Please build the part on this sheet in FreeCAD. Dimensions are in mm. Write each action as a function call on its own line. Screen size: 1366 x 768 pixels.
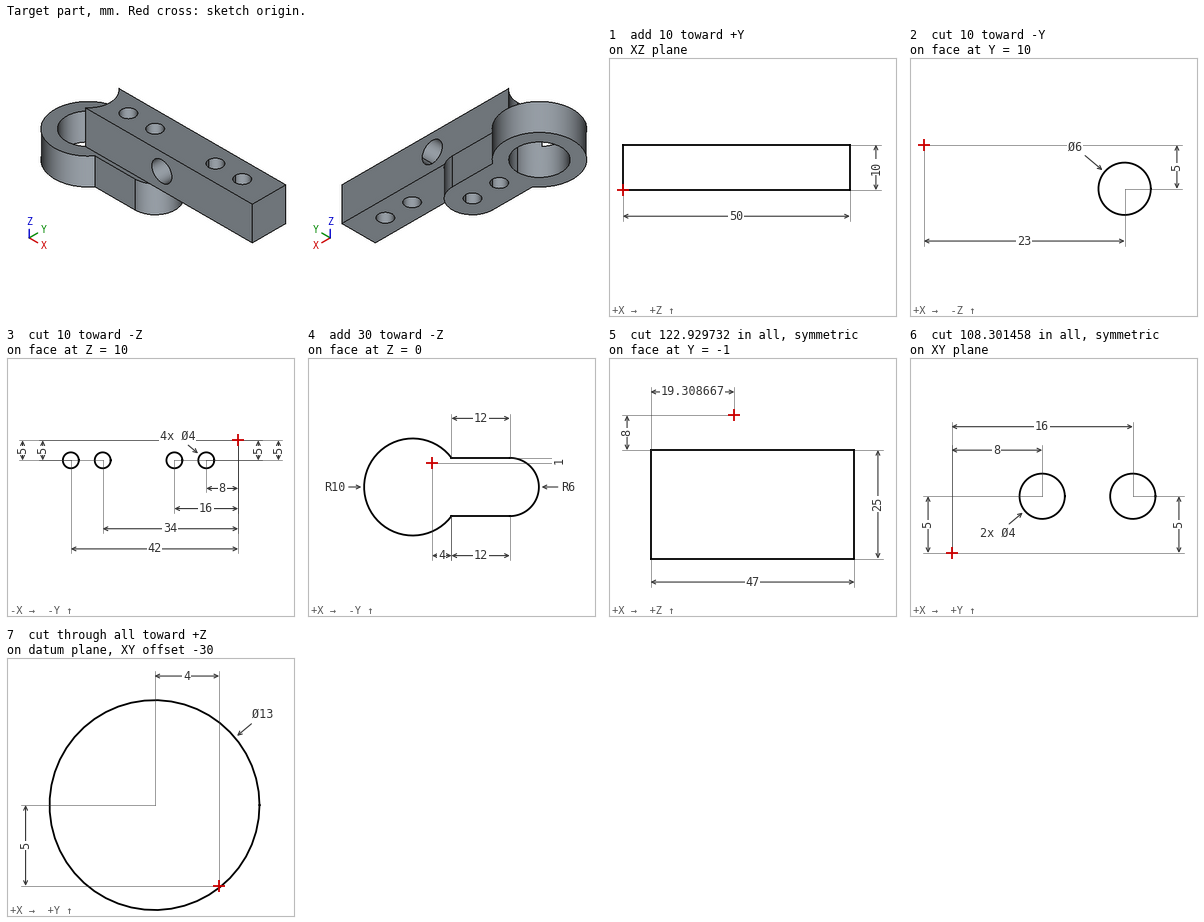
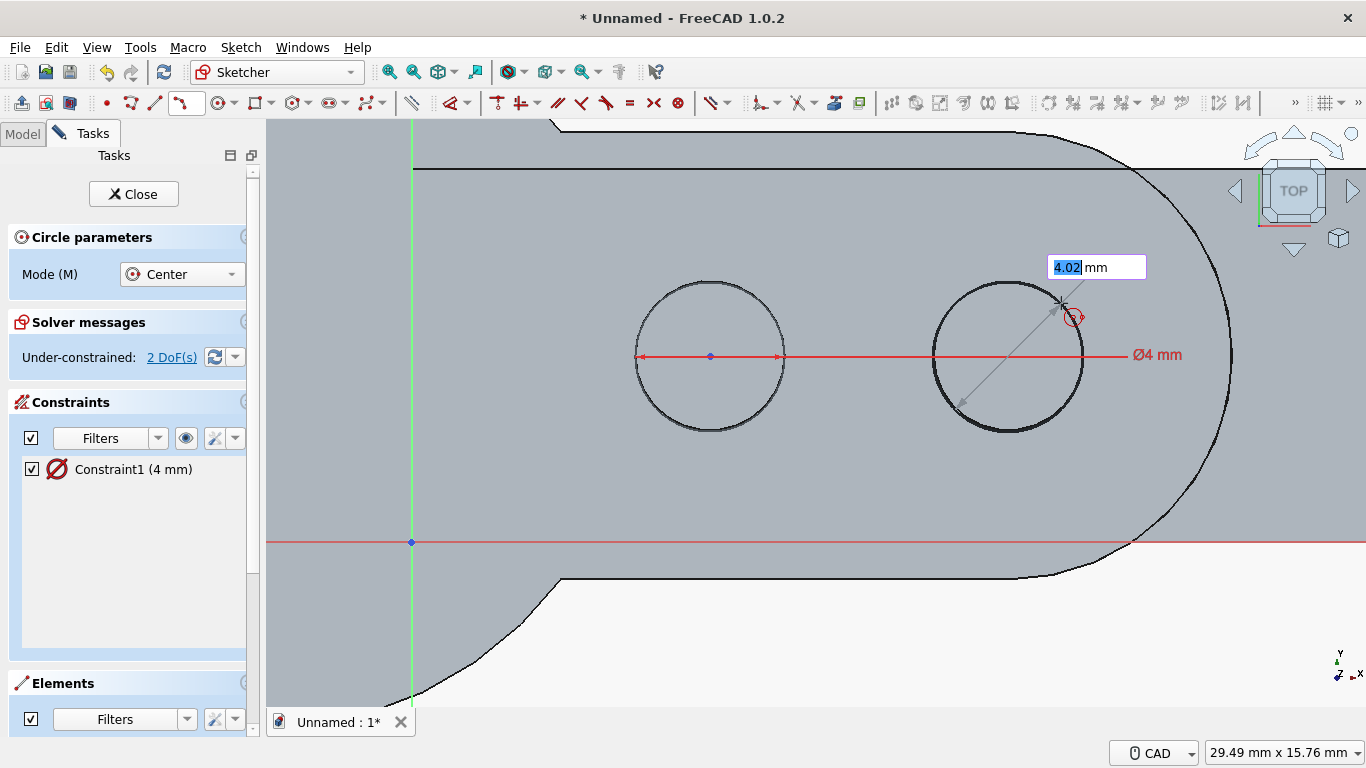
text(4)
key(Return)
key(Escape)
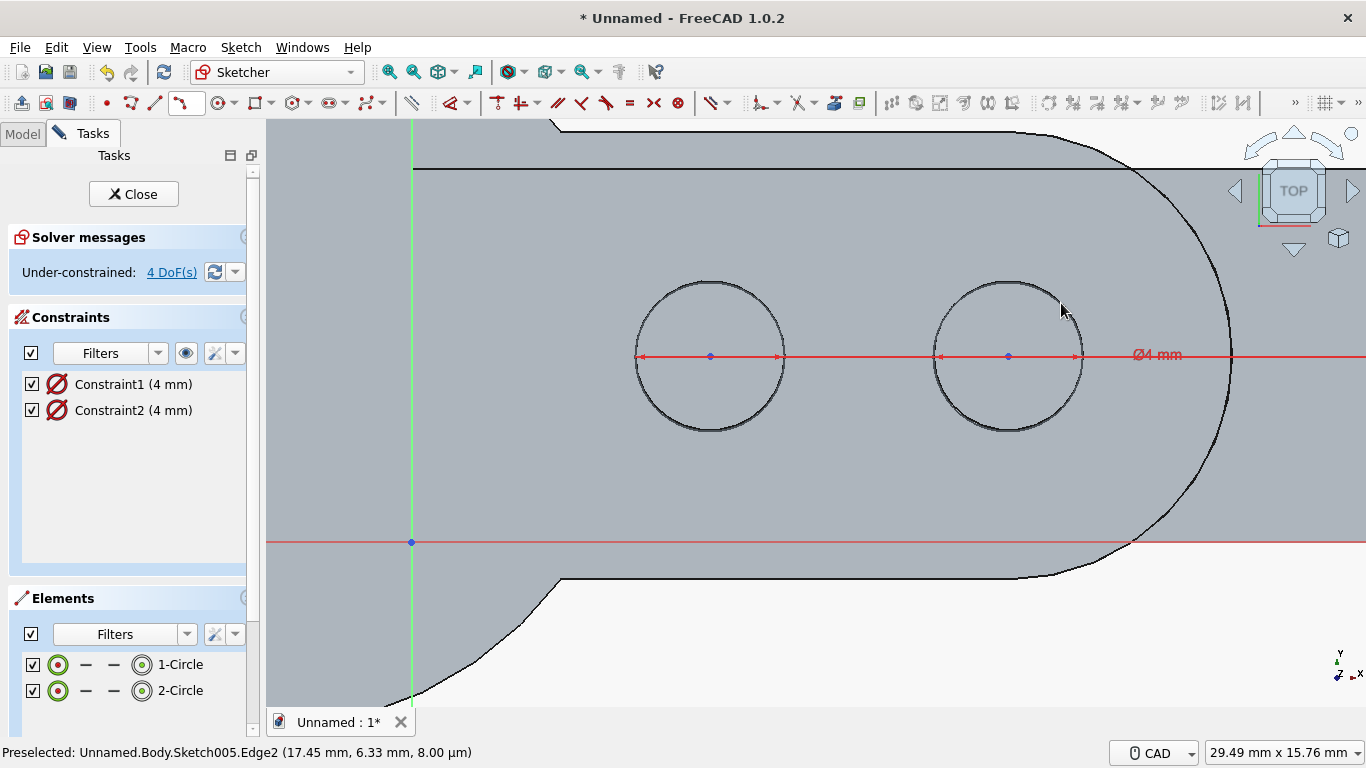
key(d)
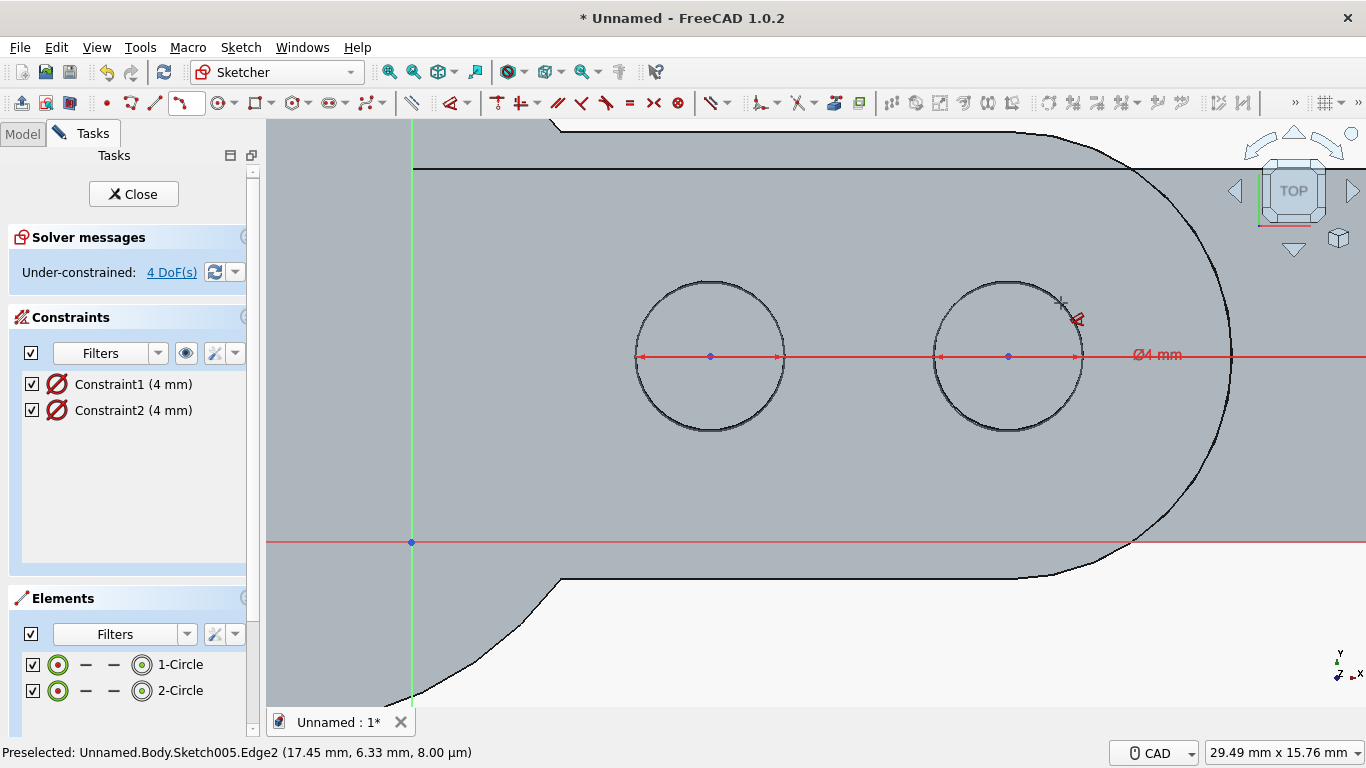
click(710, 357)
click(561, 576)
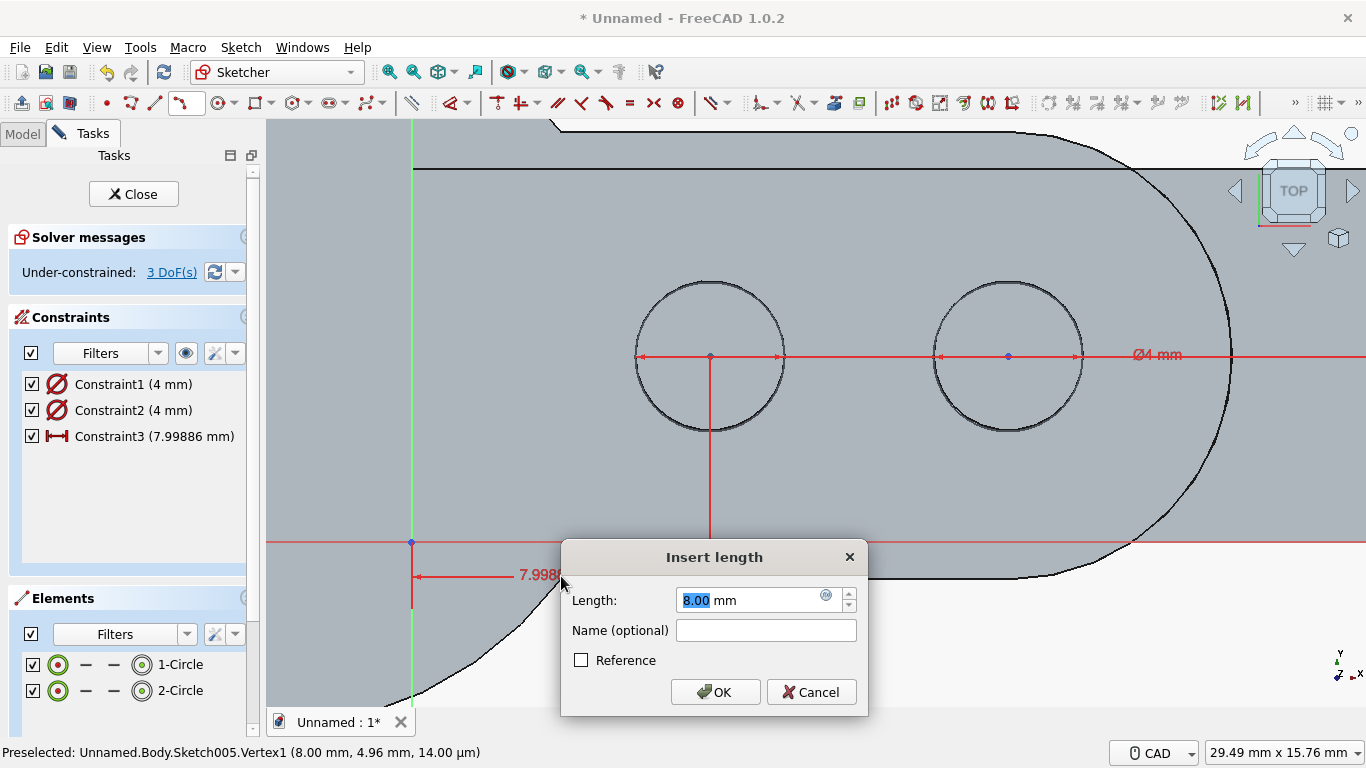
text(8)
key(Return)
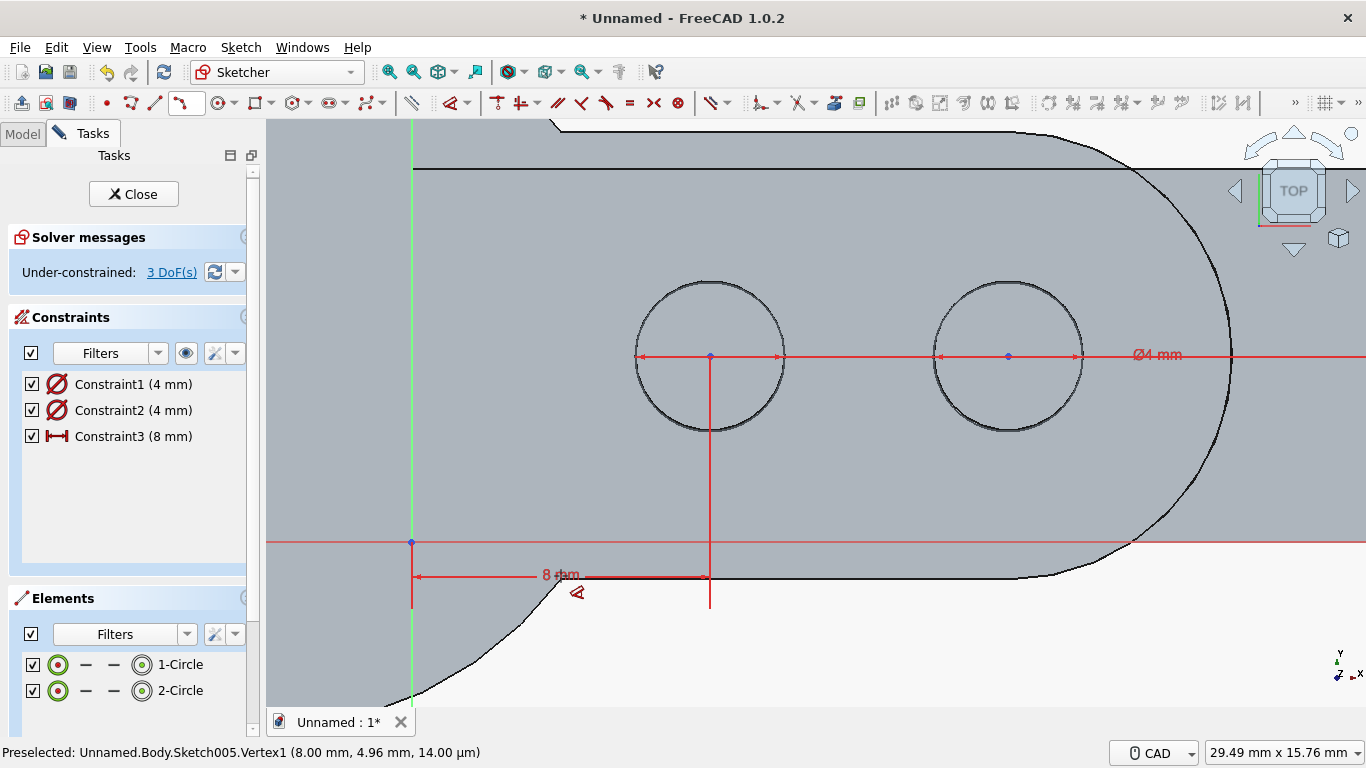
click(710, 357)
click(378, 450)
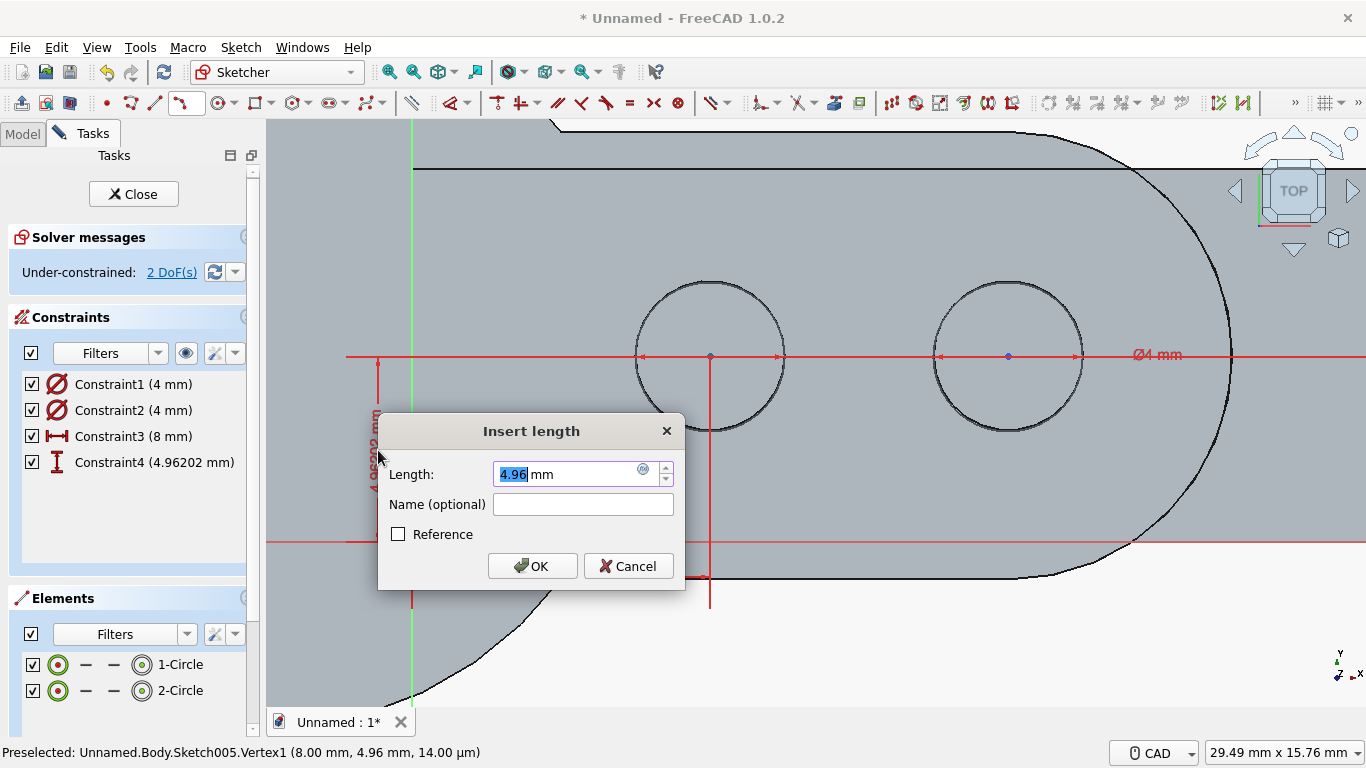
text(5)
key(Return)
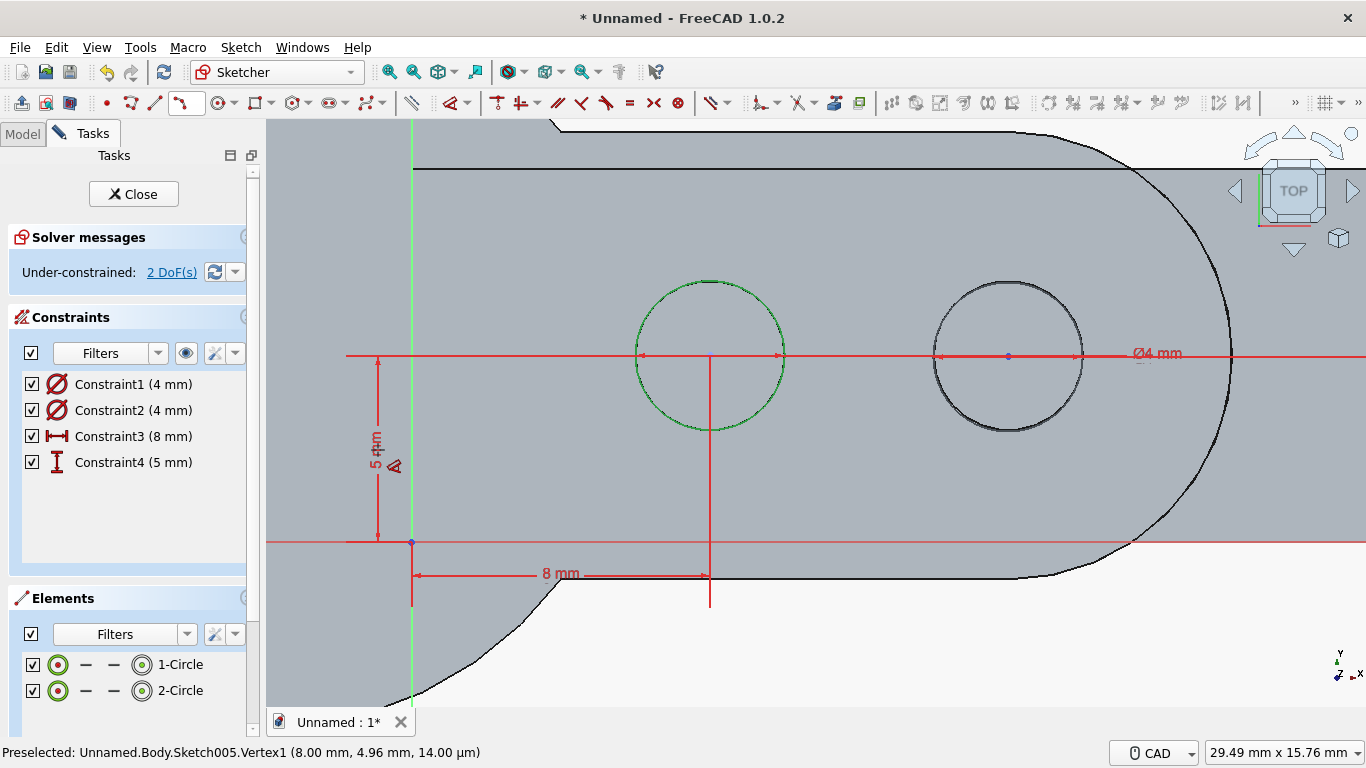
click(1008, 357)
click(378, 407)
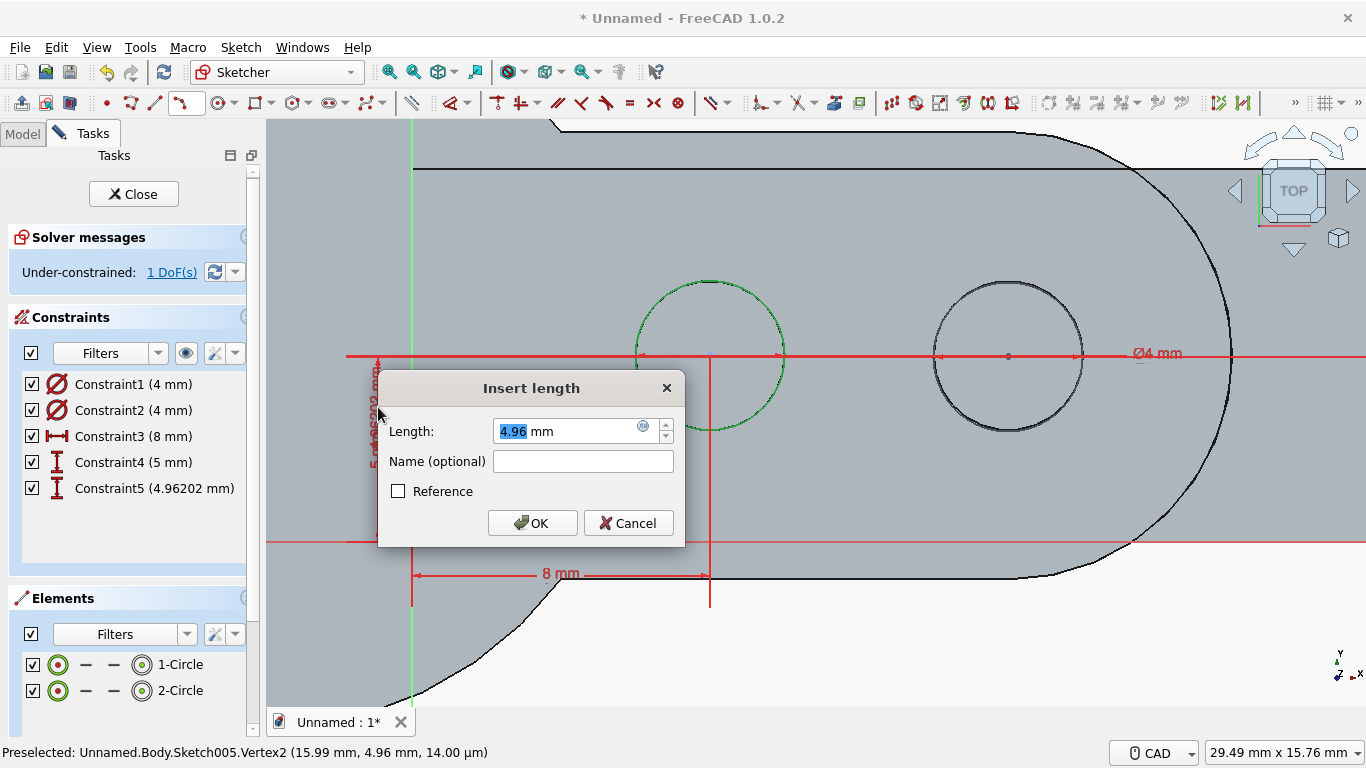
text(5)
key(Return)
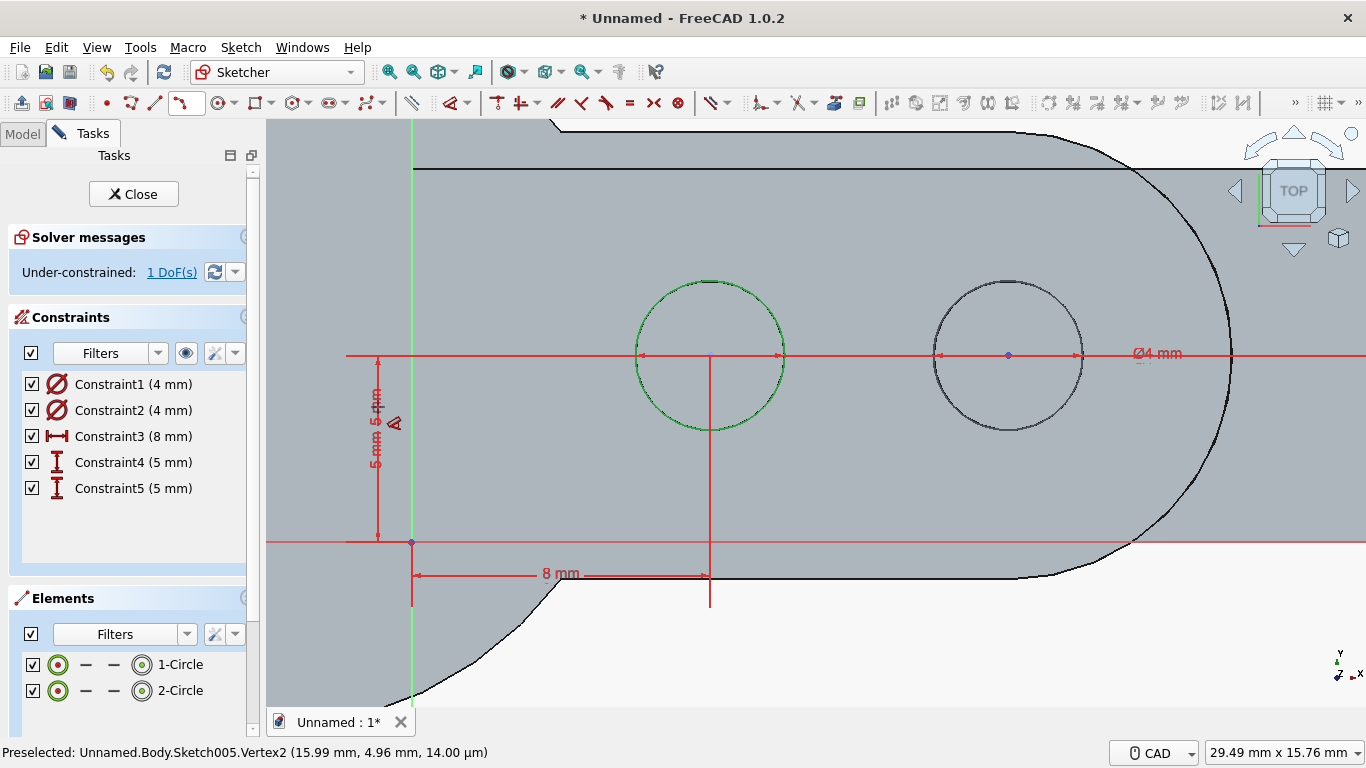
click(1008, 356)
click(710, 576)